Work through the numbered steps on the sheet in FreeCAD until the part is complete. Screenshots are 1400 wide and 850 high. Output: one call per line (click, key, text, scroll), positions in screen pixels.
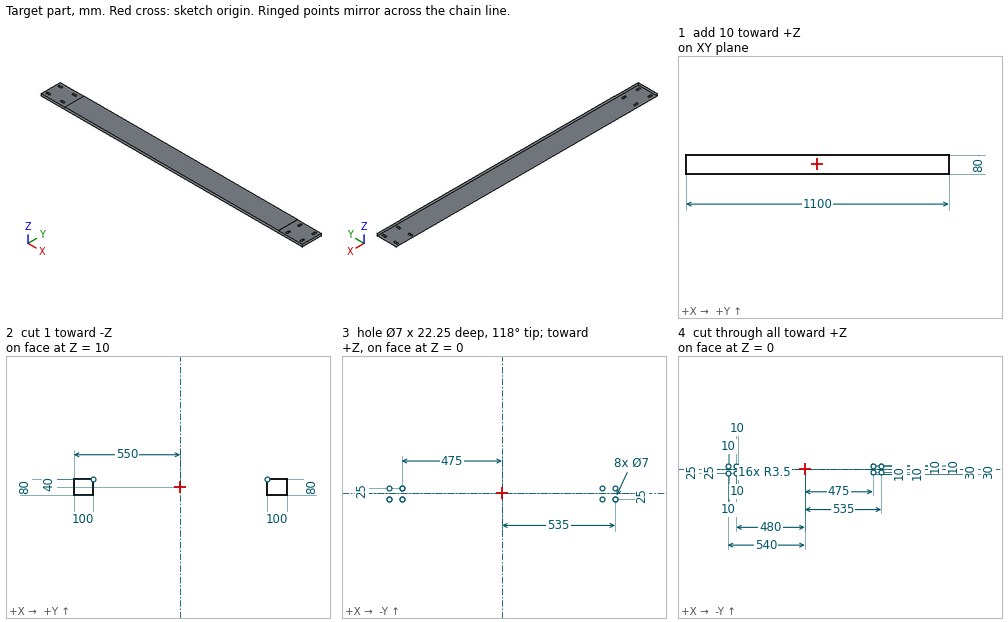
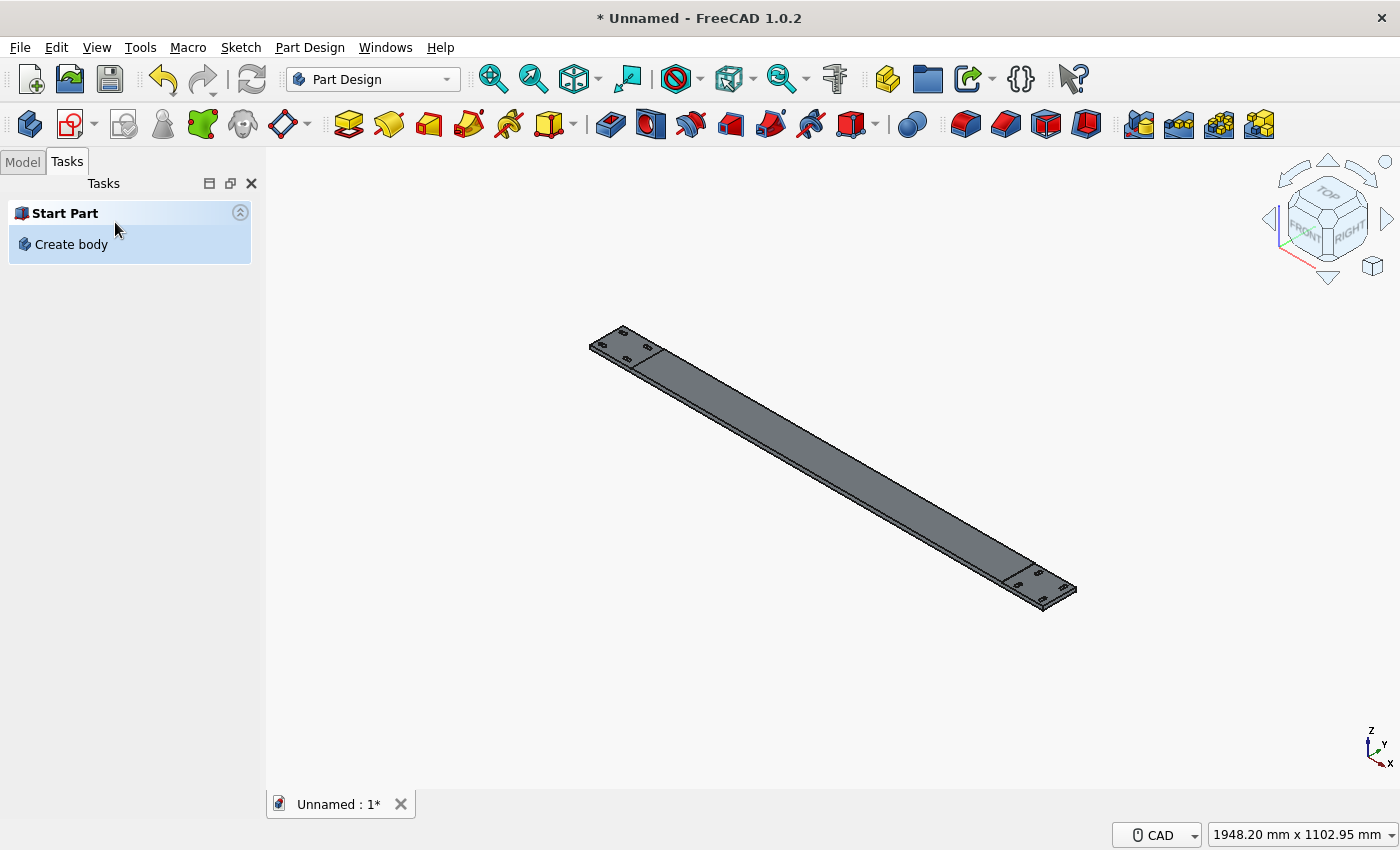
click(494, 80)